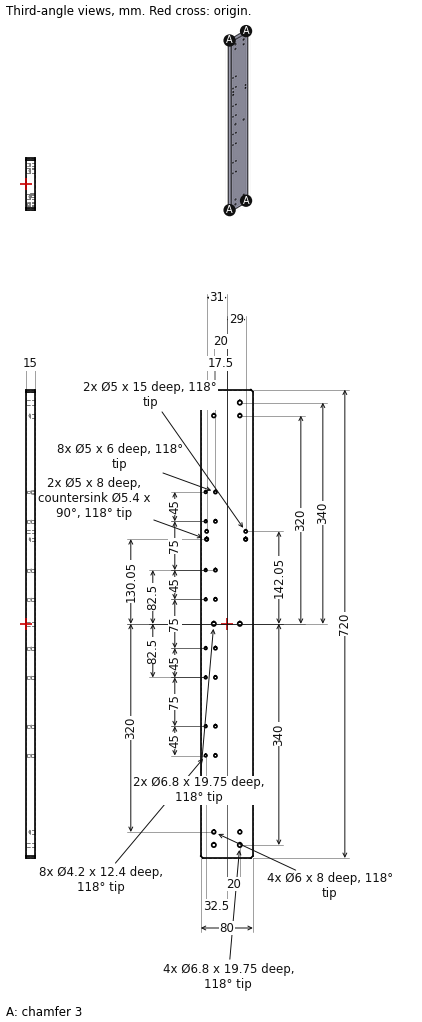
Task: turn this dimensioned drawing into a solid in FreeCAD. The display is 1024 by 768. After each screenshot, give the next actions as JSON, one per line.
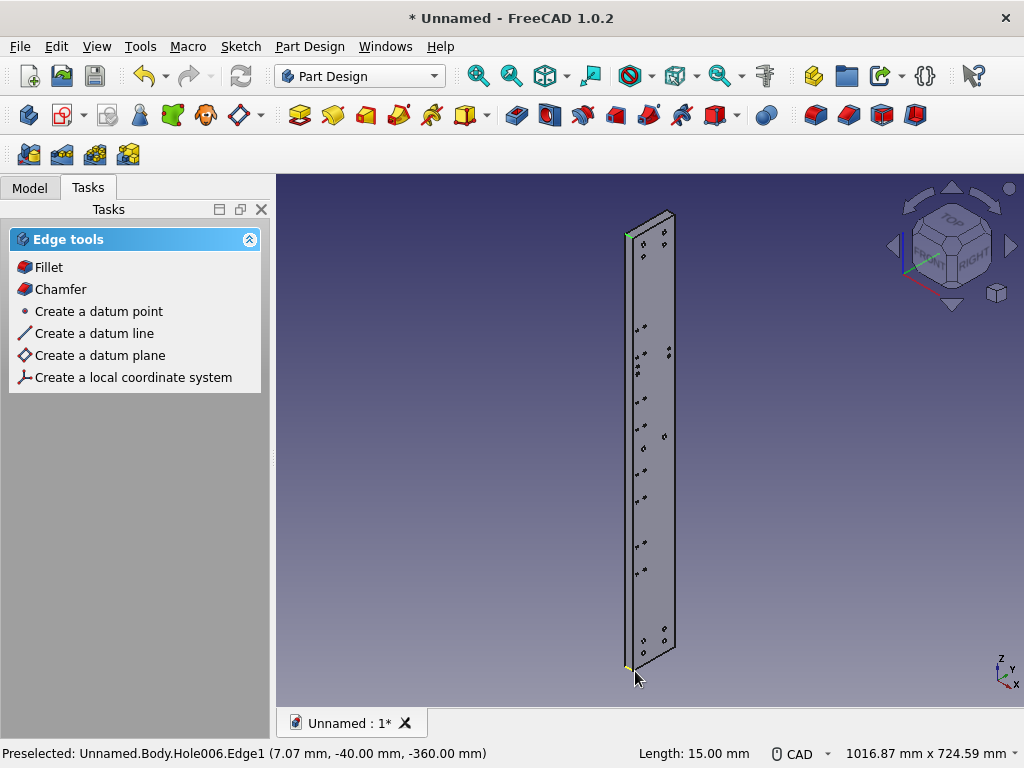
{"action": "scroll", "coordinate": [629, 668], "scroll_direction": "up", "scroll_amount": 7}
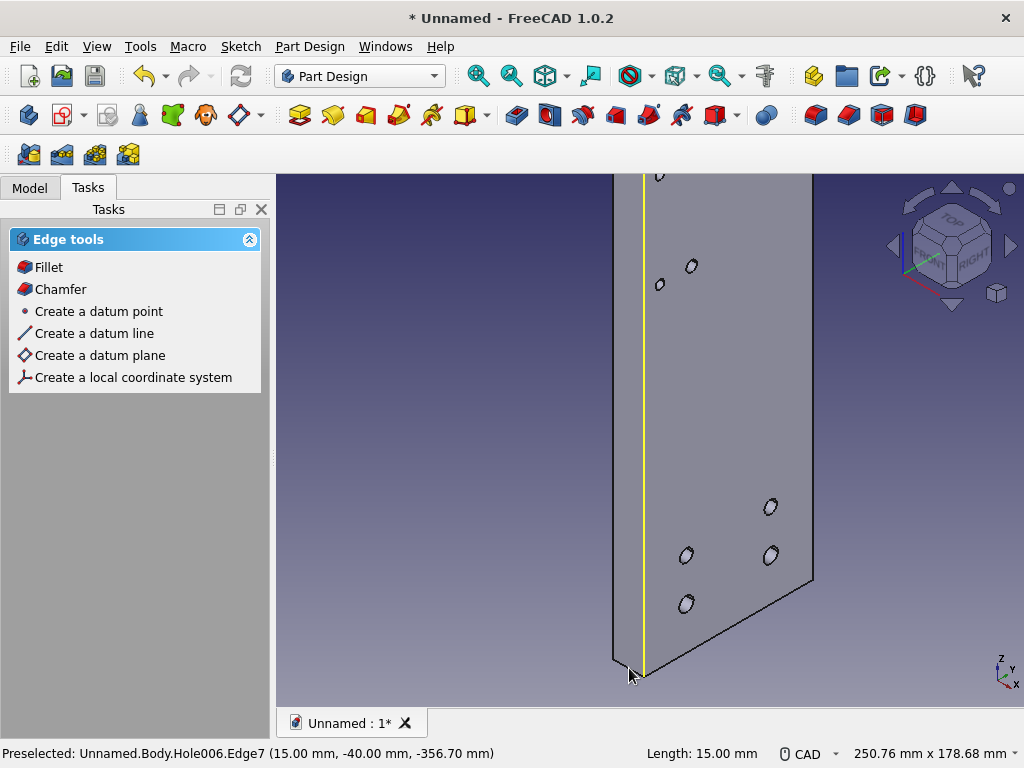
{"action": "left_click", "coordinate": [479, 76]}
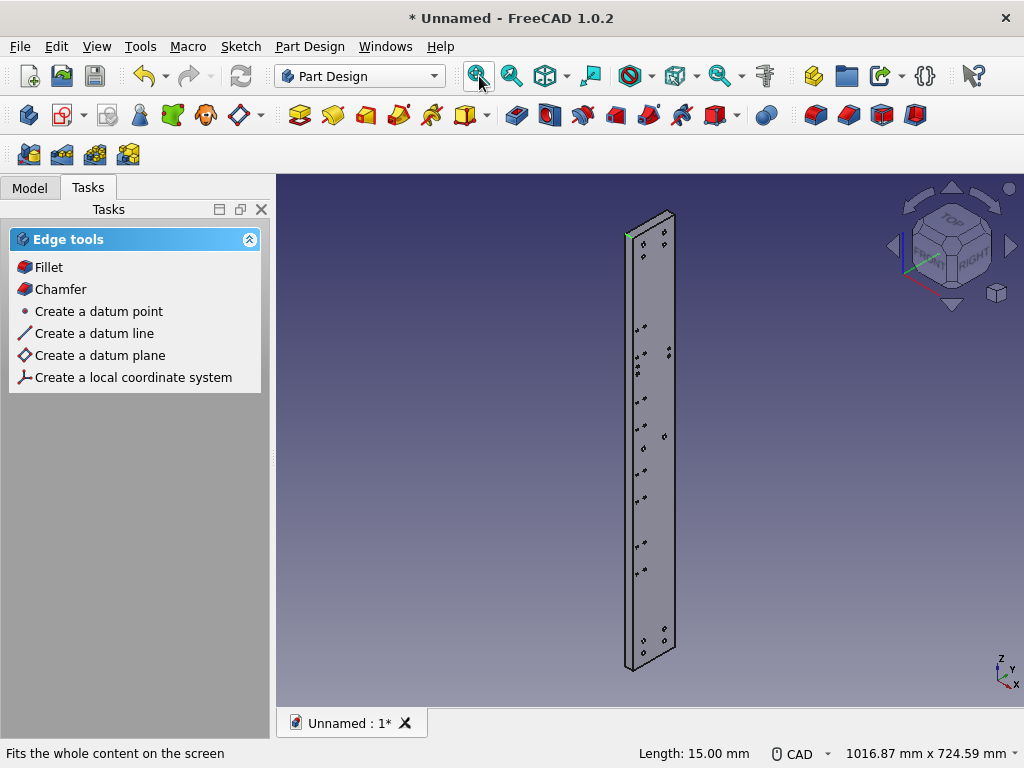
{"action": "key", "text": "2"}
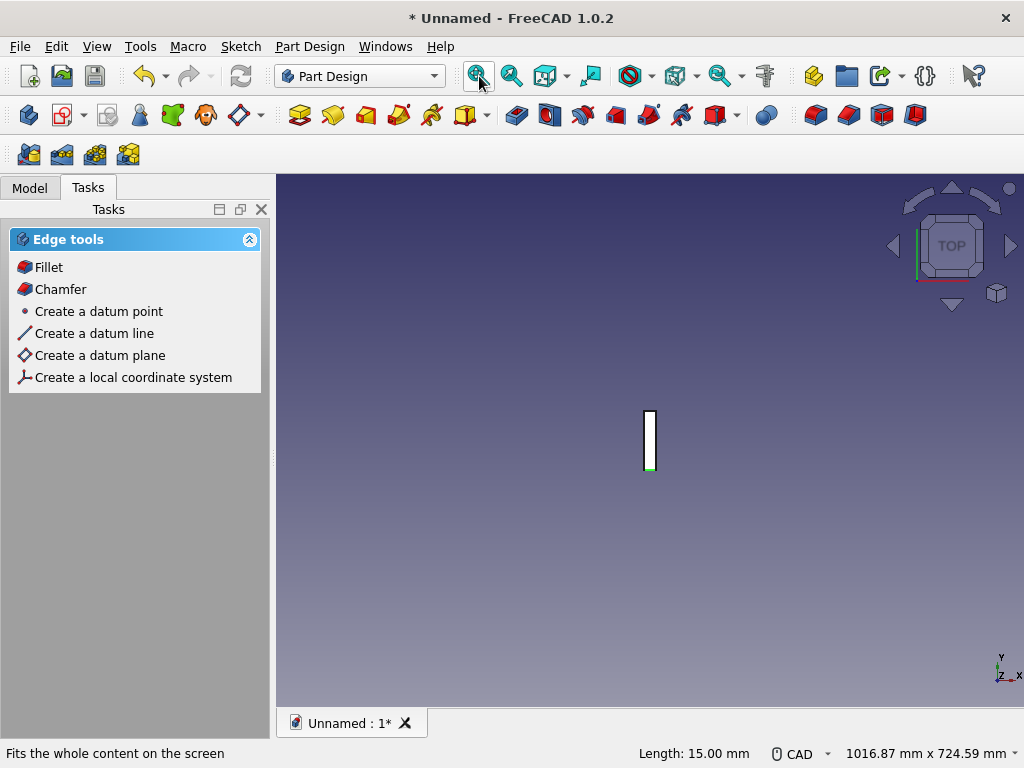
{"action": "left_click", "coordinate": [479, 76]}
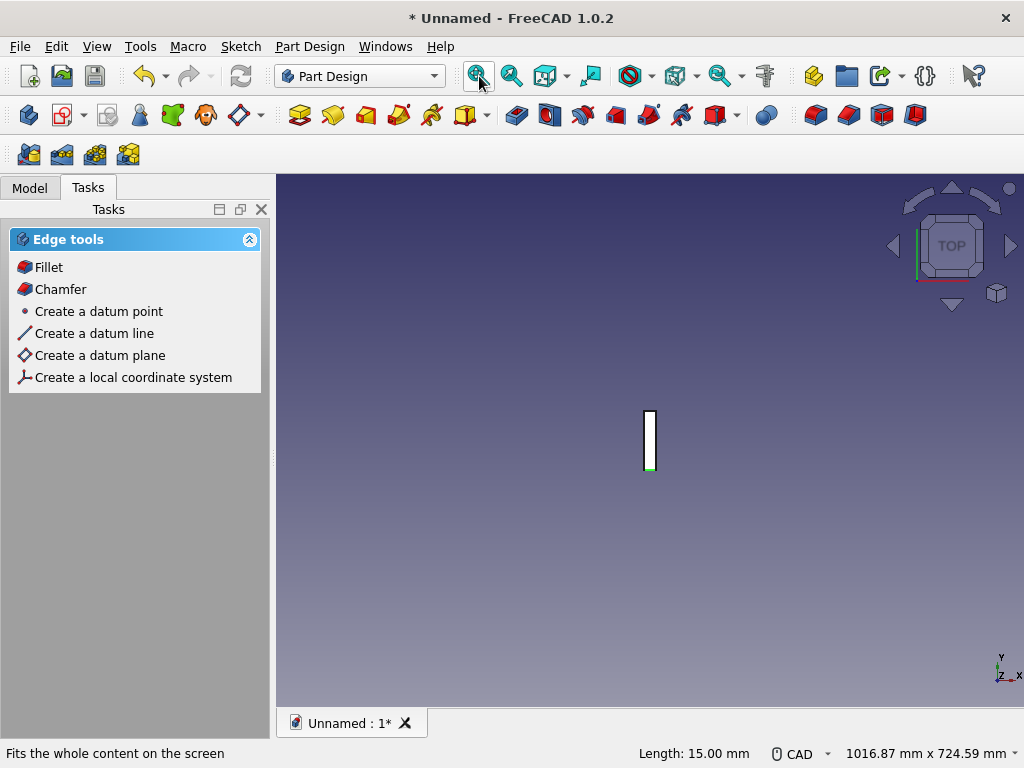
{"action": "scroll", "coordinate": [650, 469], "scroll_direction": "up", "scroll_amount": 7}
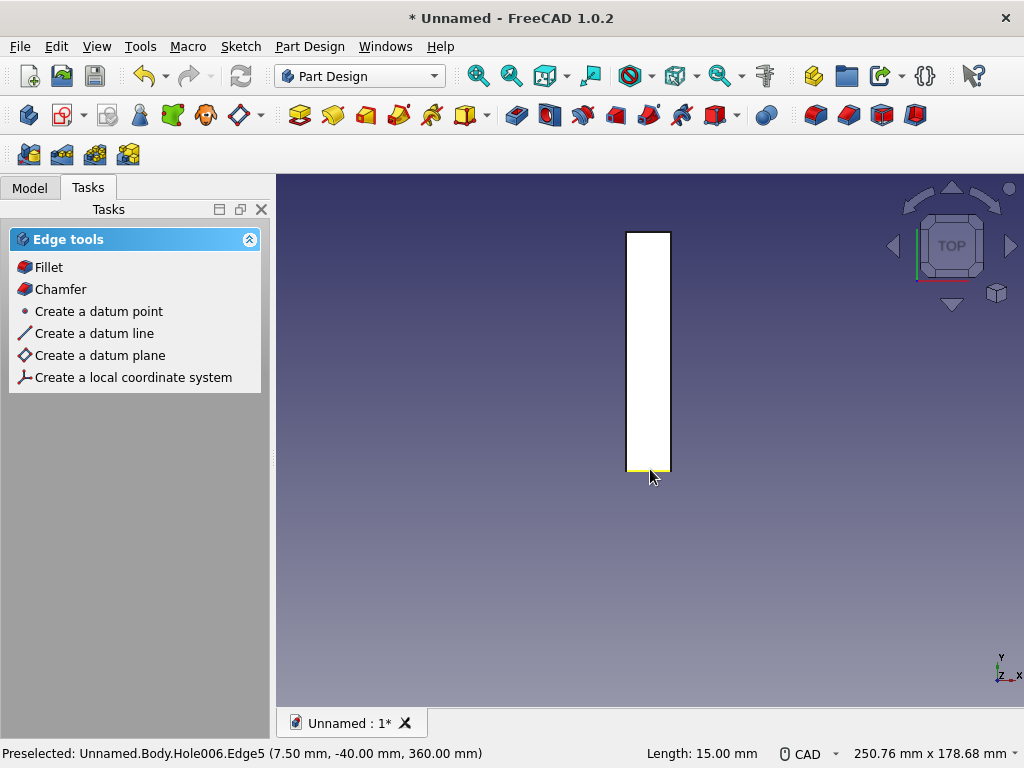
{"action": "left_click", "coordinate": [648, 231], "text": "ctrl"}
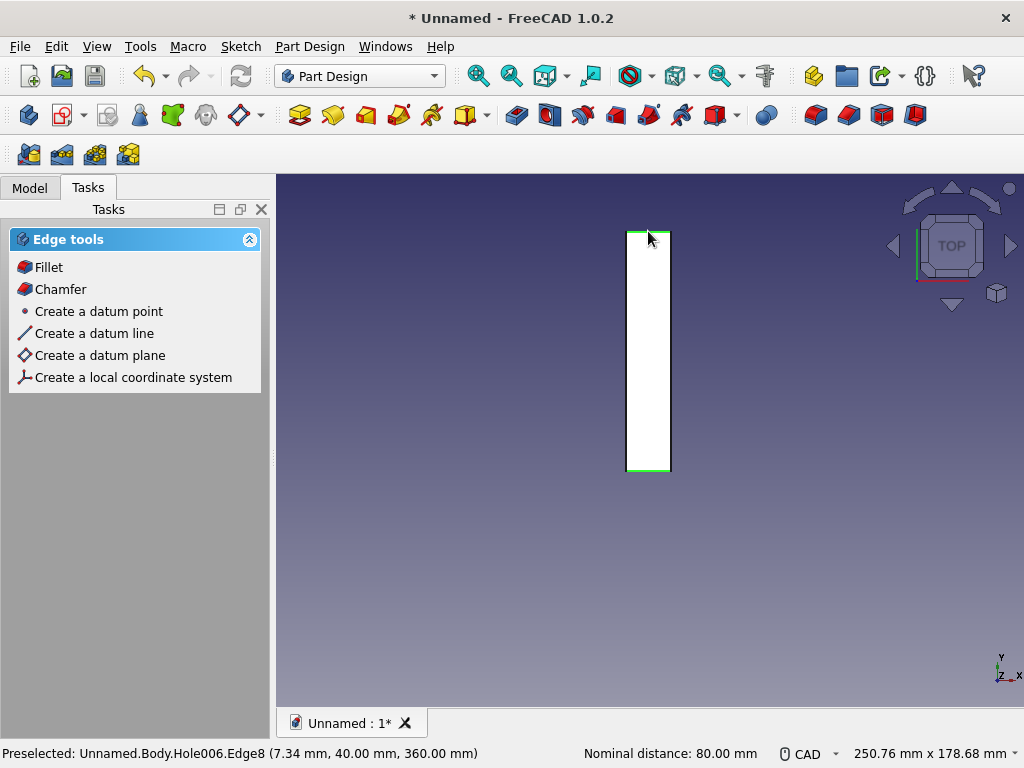
{"action": "left_click", "coordinate": [479, 76]}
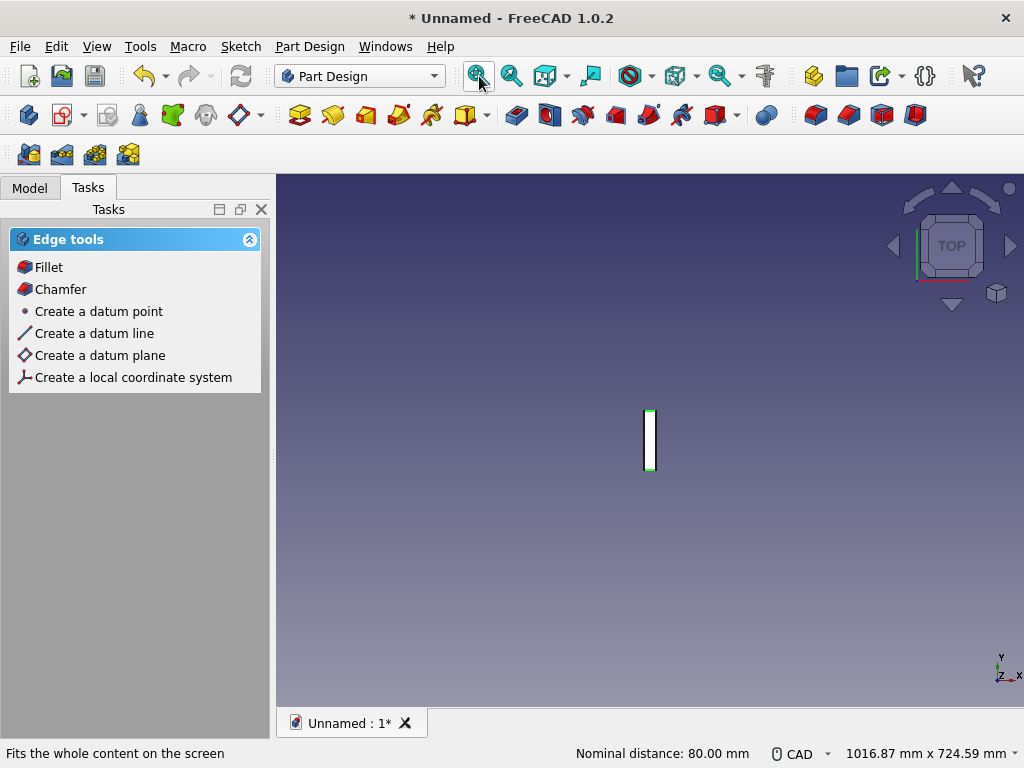
{"action": "key", "text": "1"}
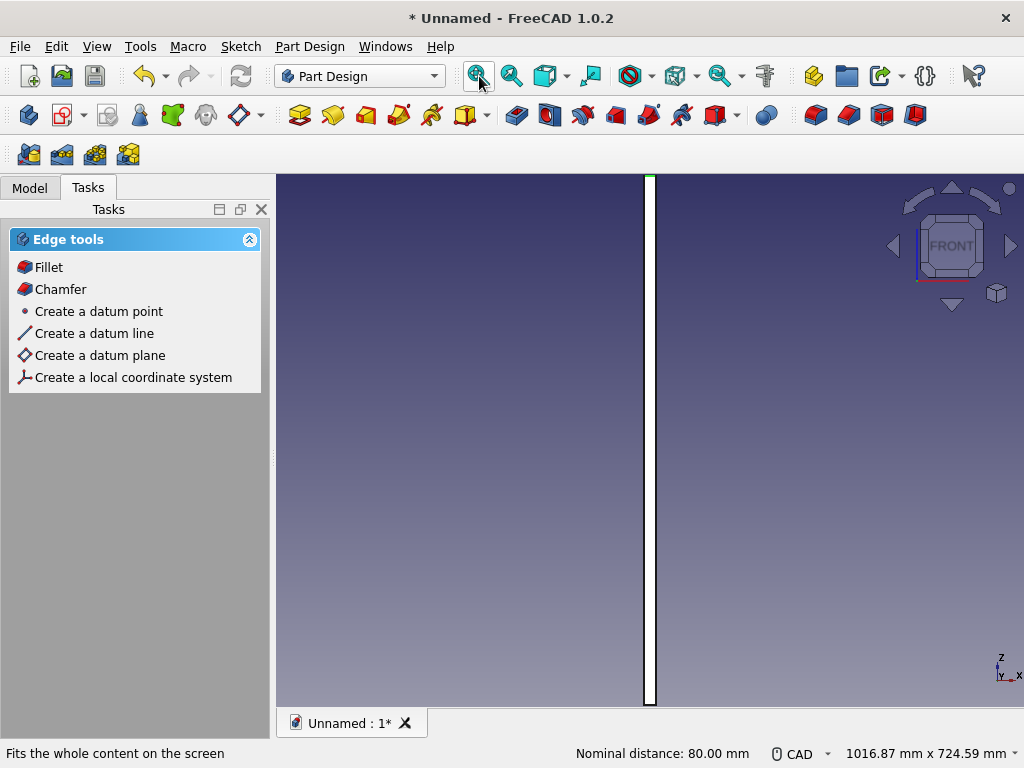
{"action": "key", "text": "3"}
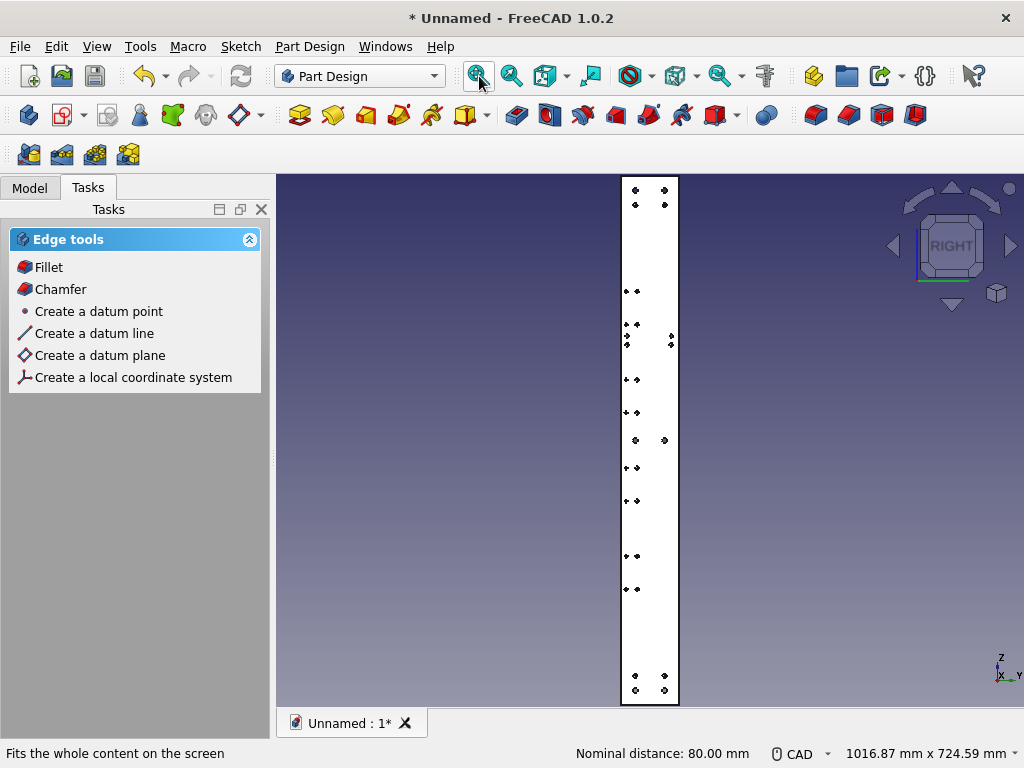
{"action": "key", "text": "5"}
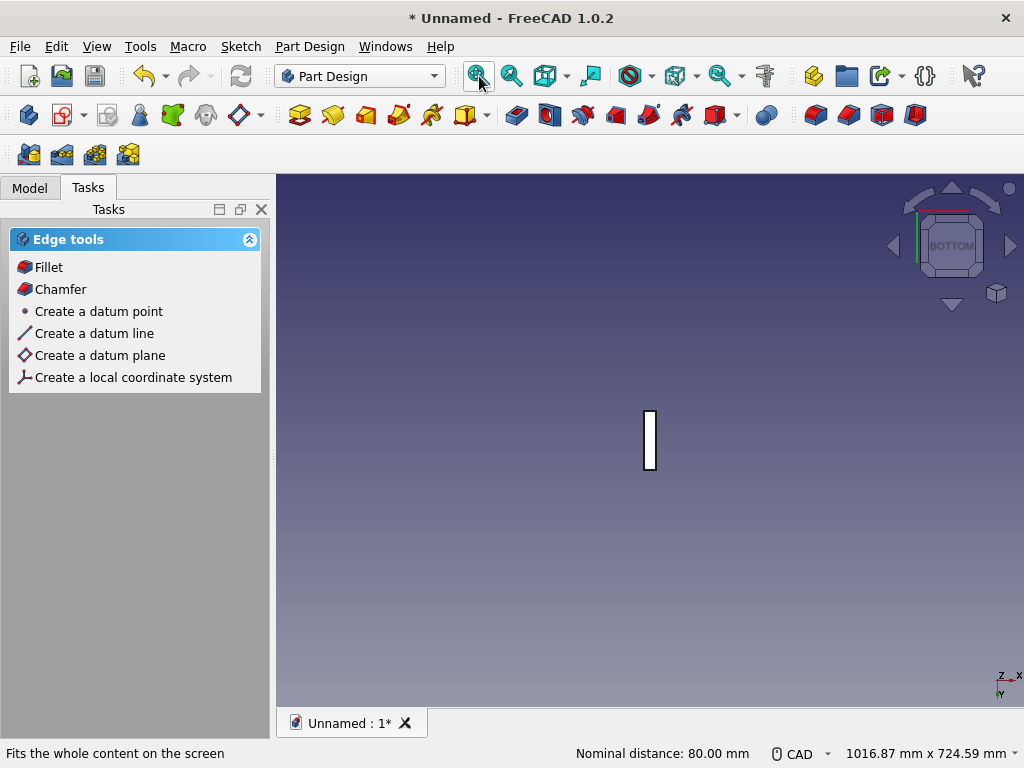
{"action": "left_click", "coordinate": [479, 76]}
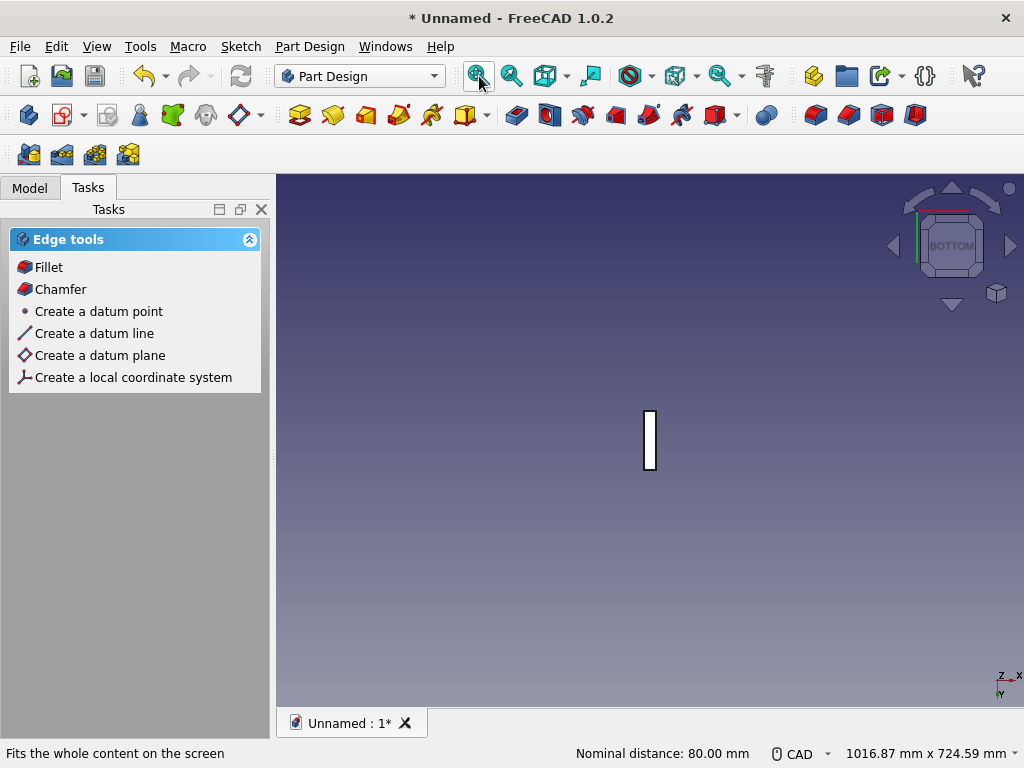
{"action": "scroll", "coordinate": [650, 410], "scroll_direction": "up", "scroll_amount": 7}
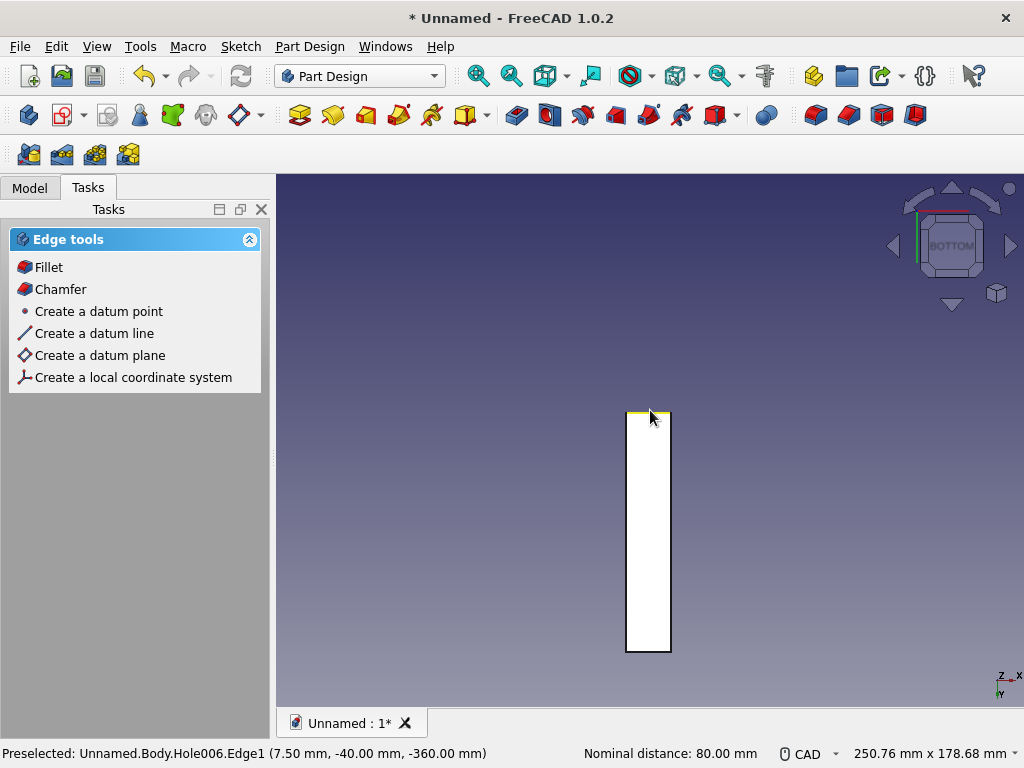
{"action": "left_click", "coordinate": [648, 412], "text": "ctrl"}